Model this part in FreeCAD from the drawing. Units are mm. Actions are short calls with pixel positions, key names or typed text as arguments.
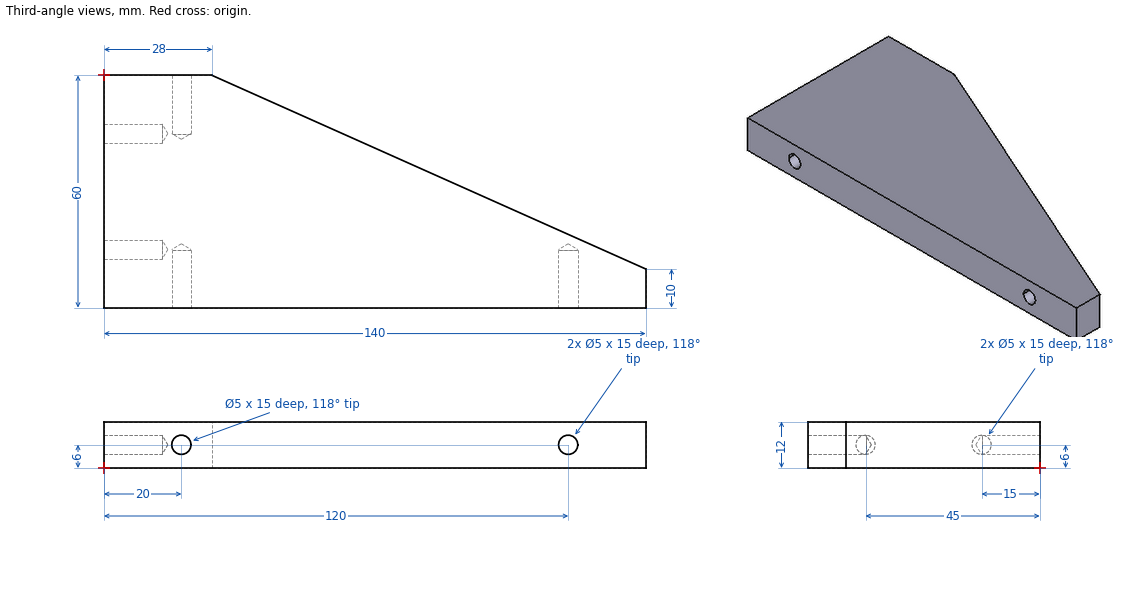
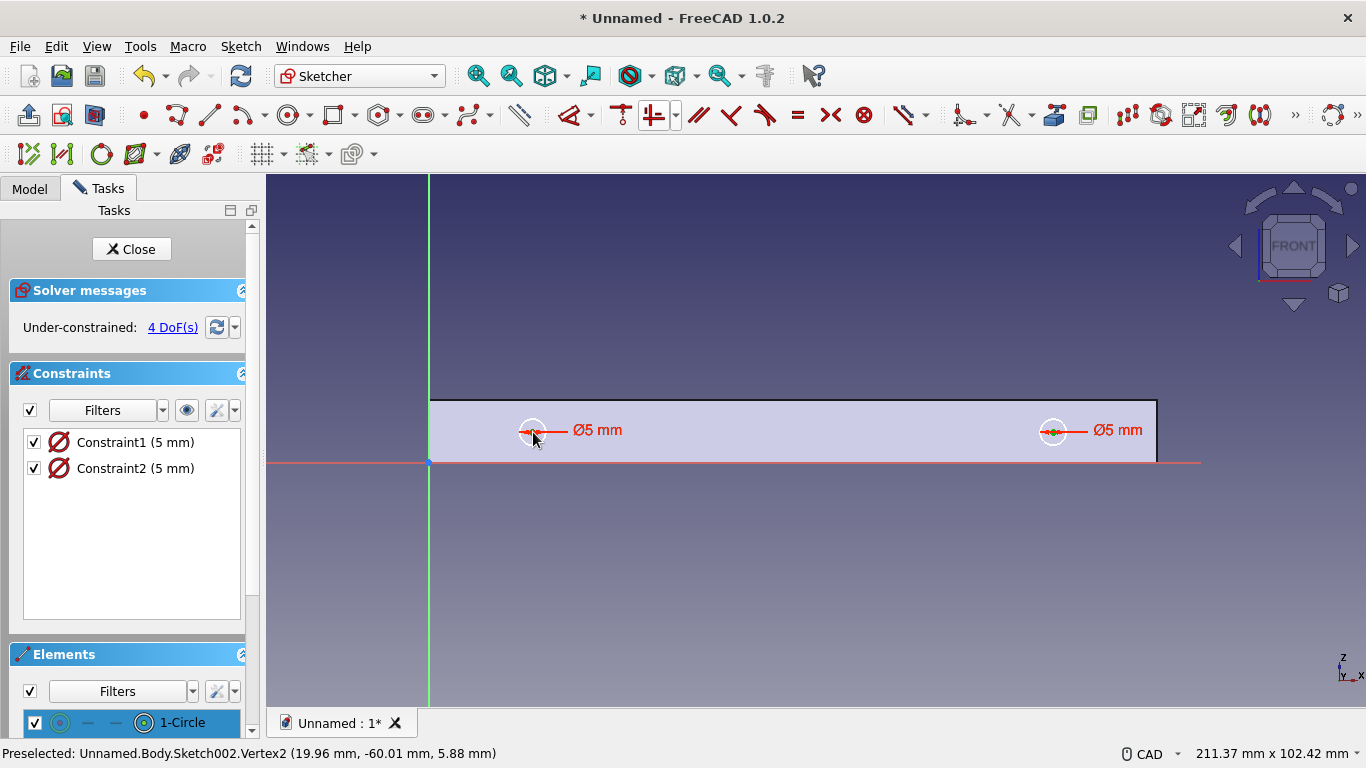
key(h)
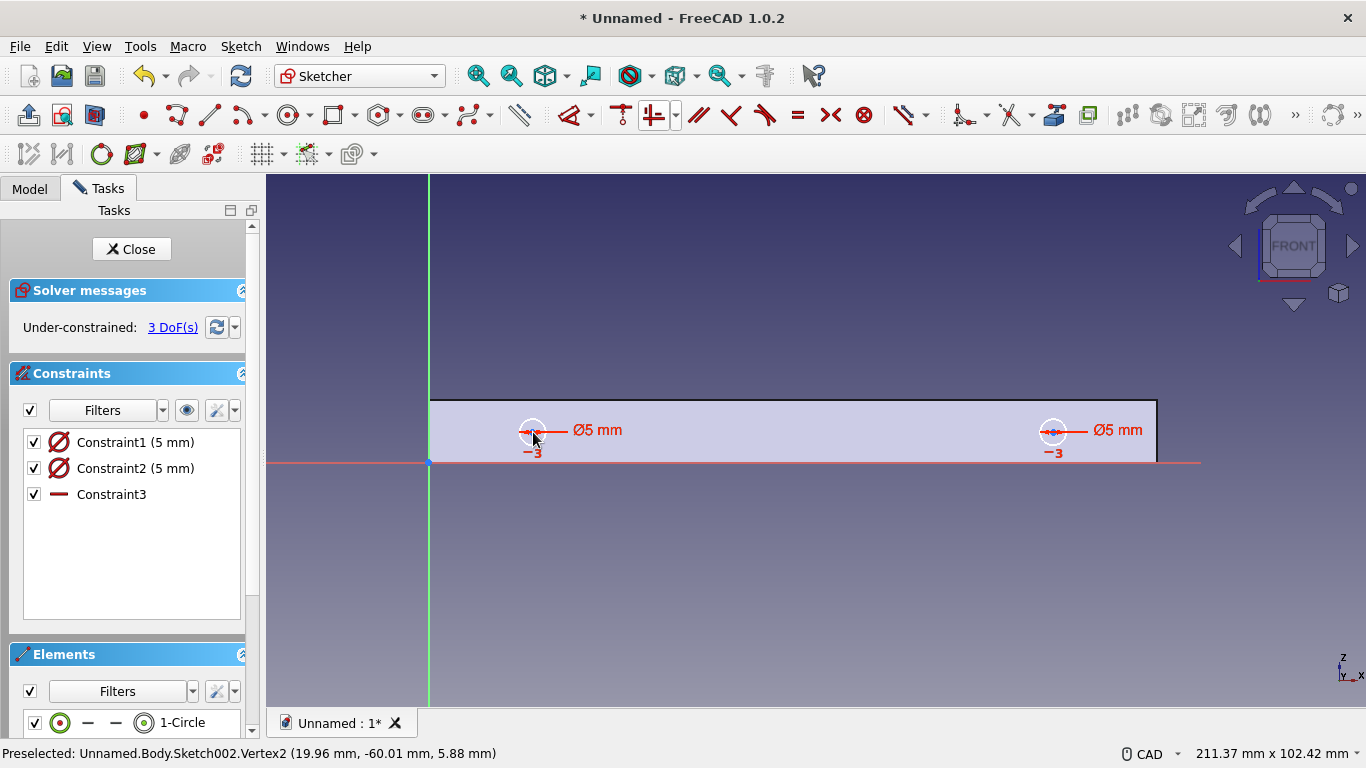
click(568, 116)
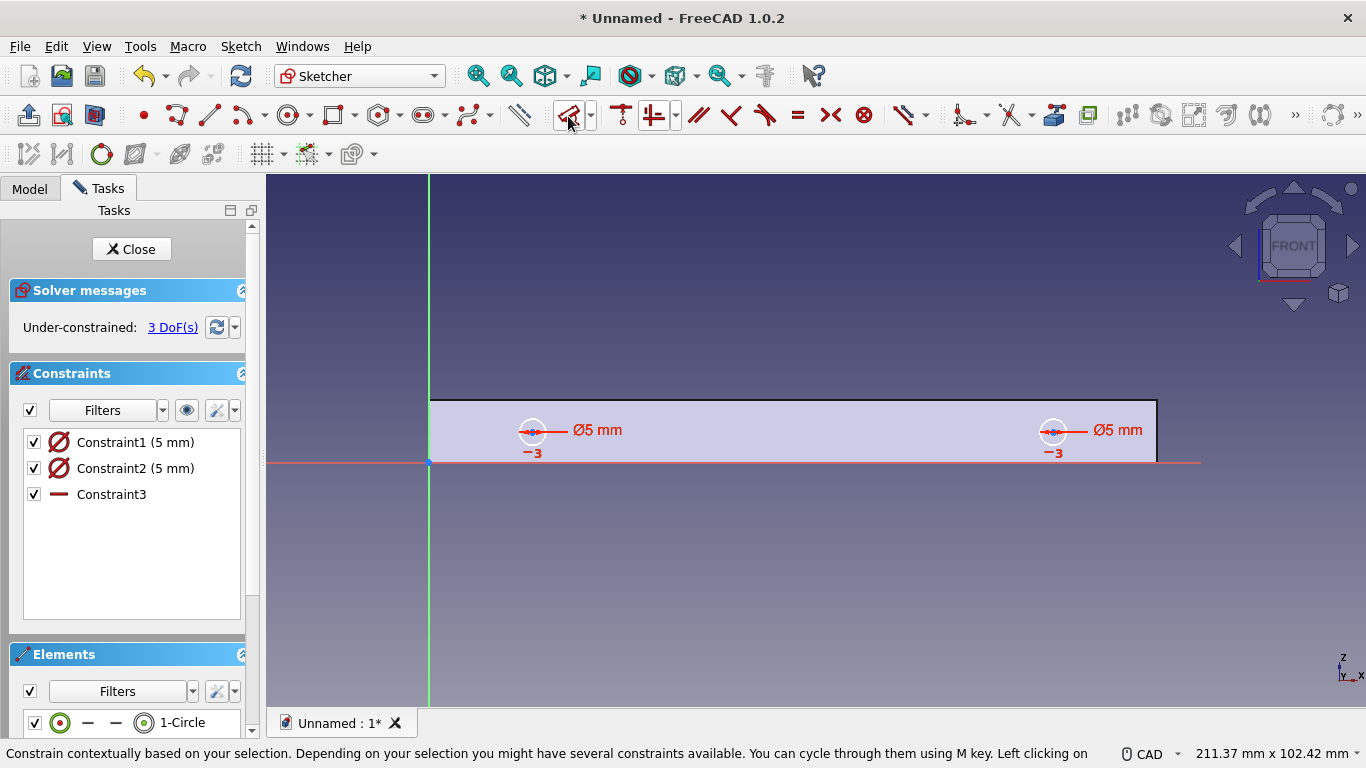
scroll(1053, 432, up, 2)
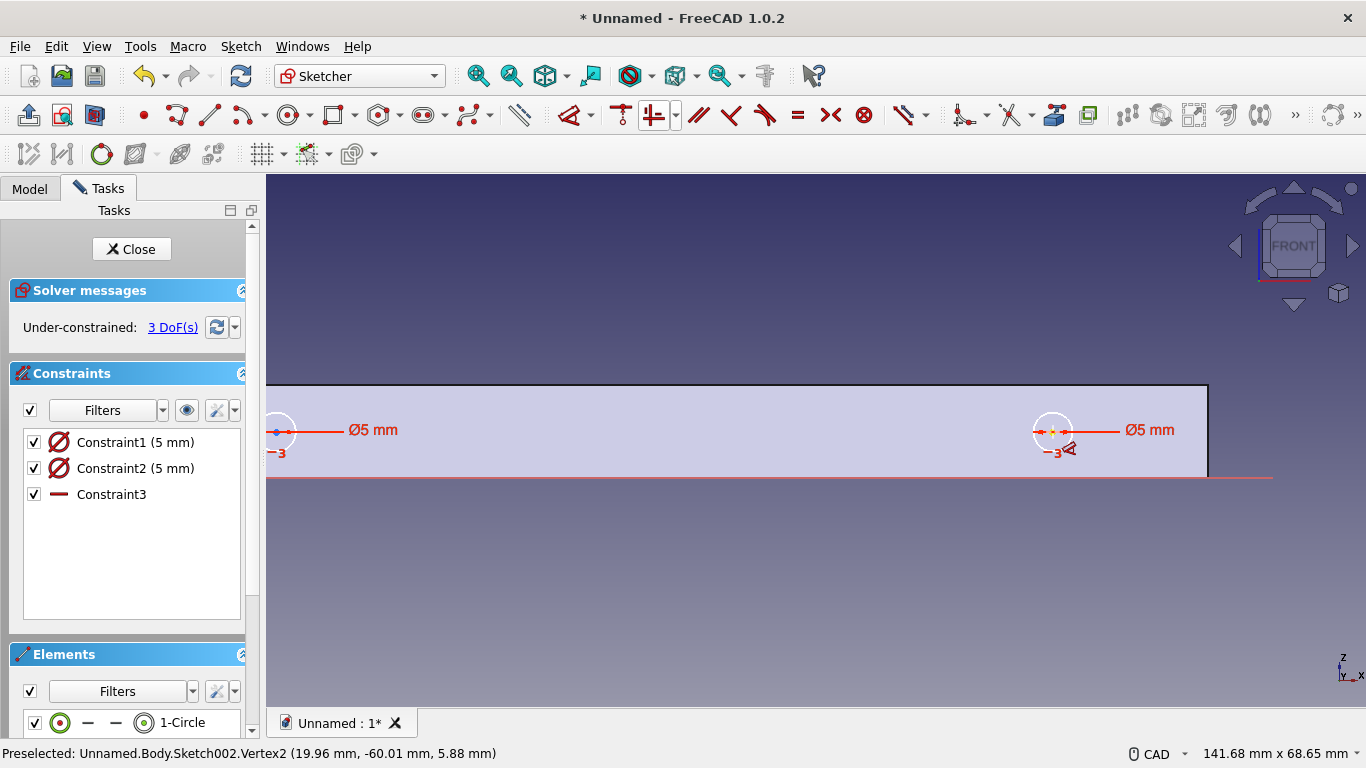
click(1053, 432)
click(1087, 455)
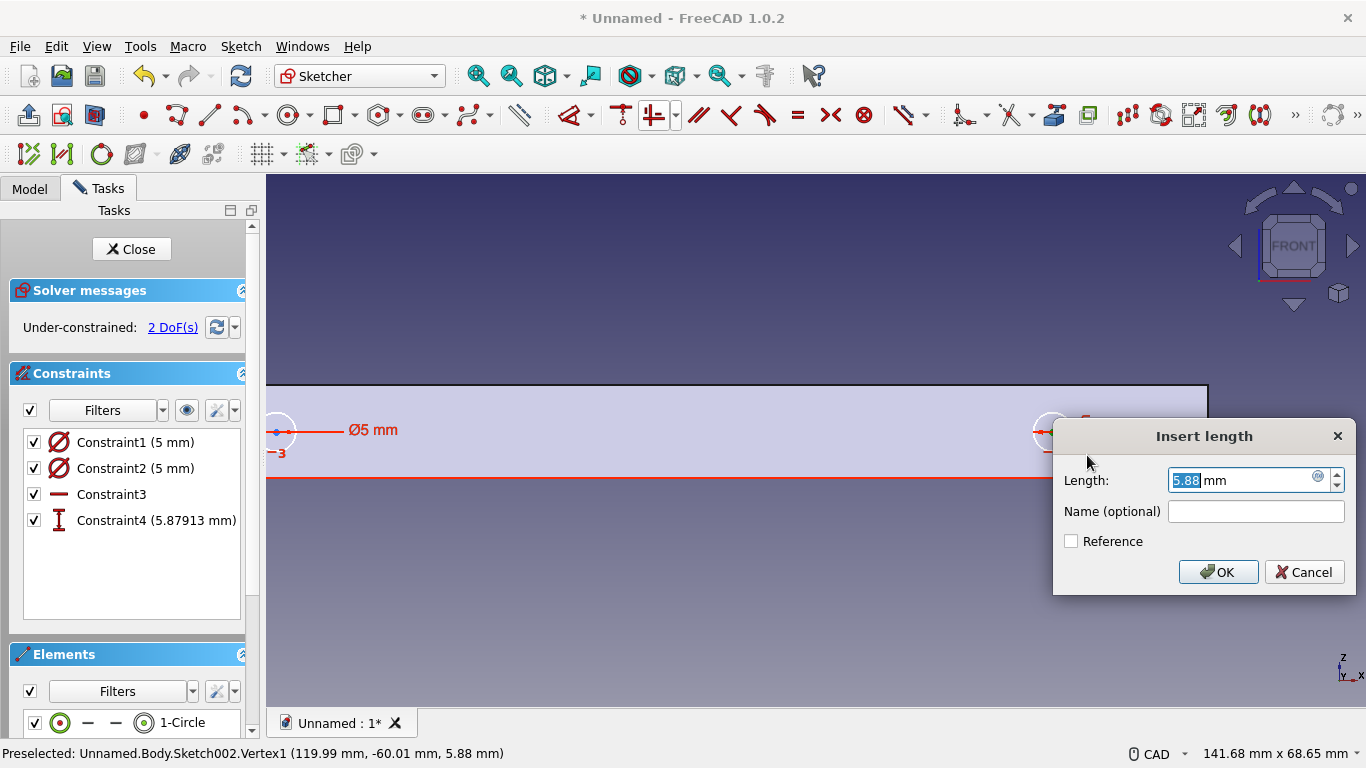
text(6)
key(Return)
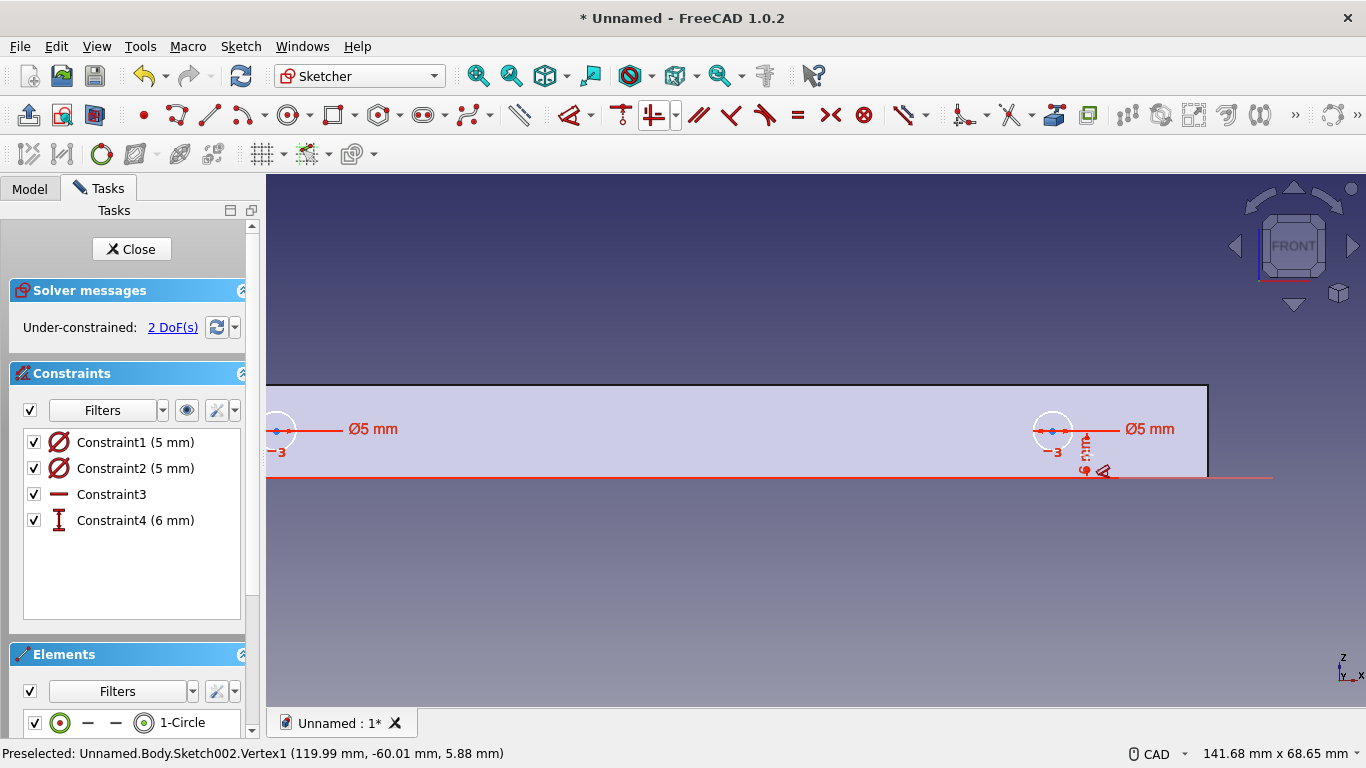
scroll(1054, 432, down, 2)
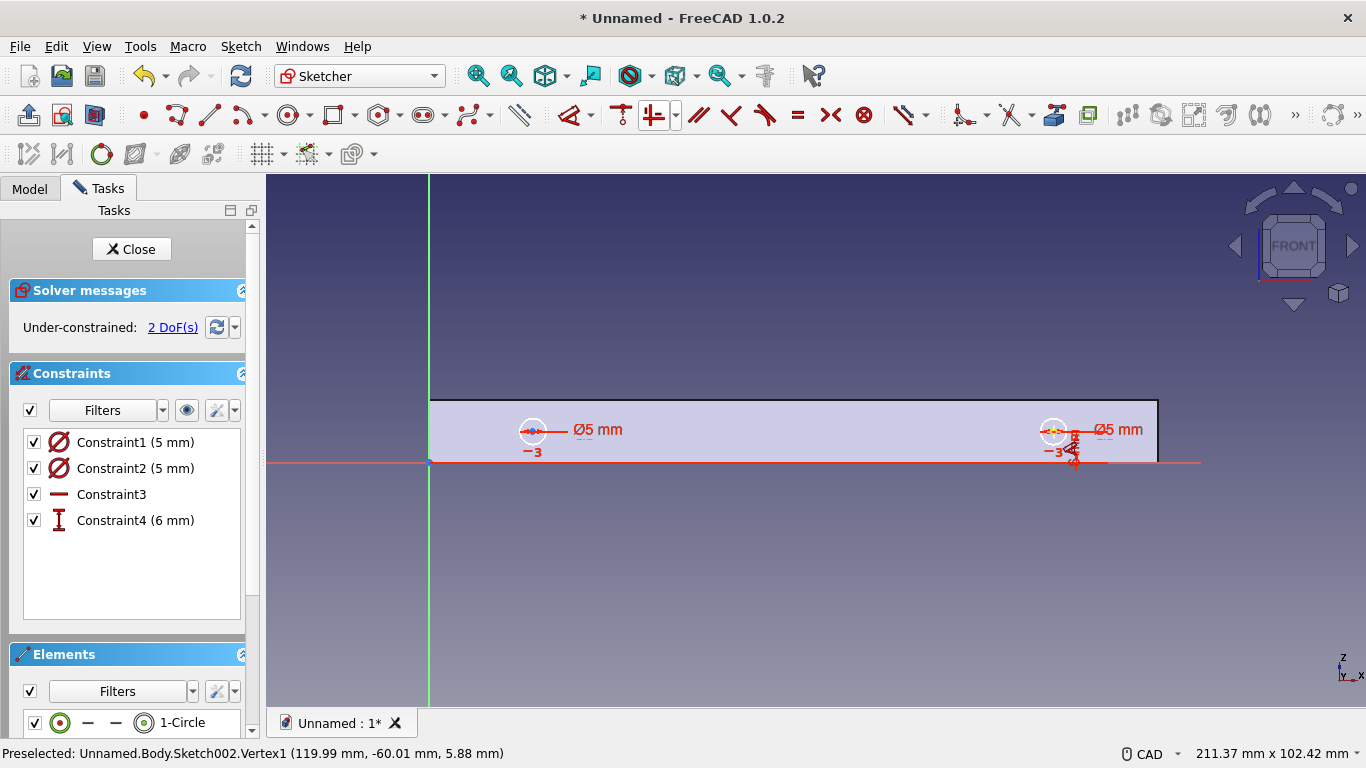
click(533, 432)
click(481, 497)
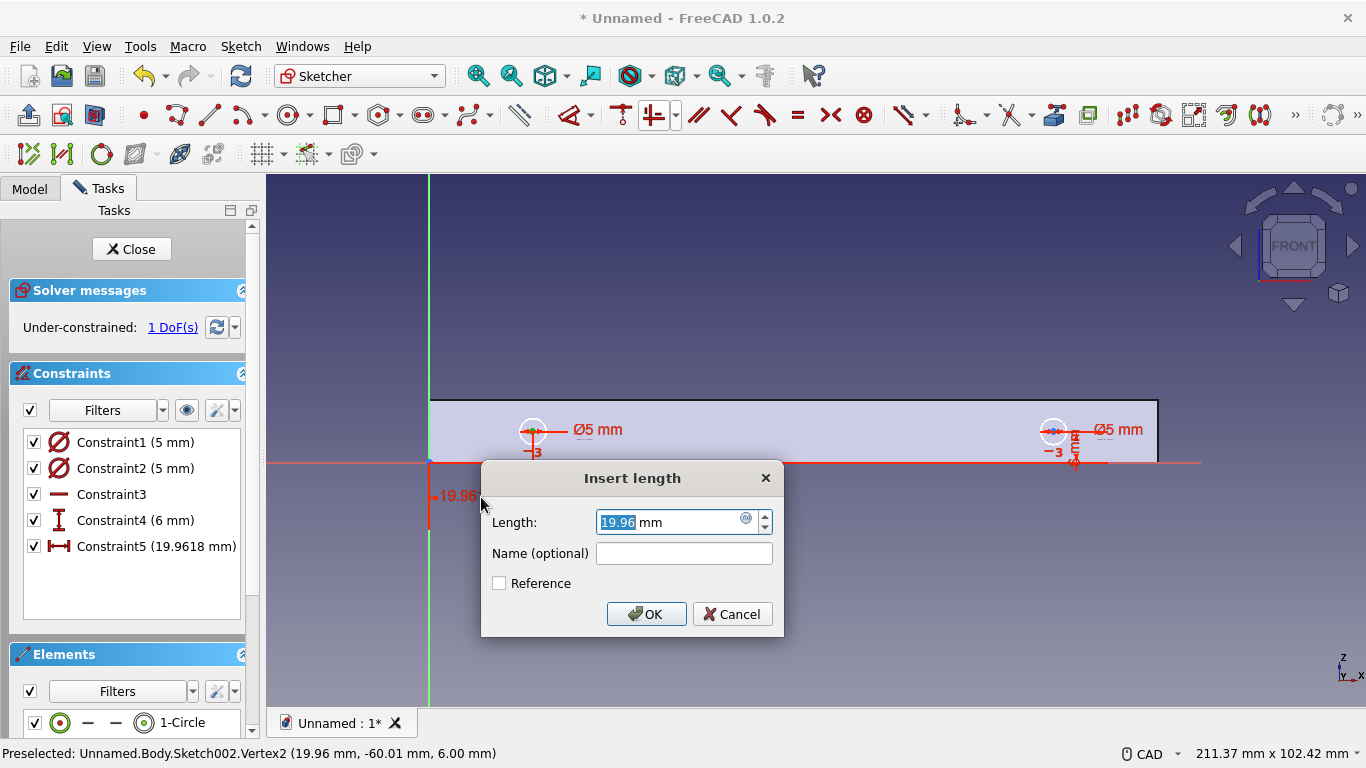
text(20)
key(Return)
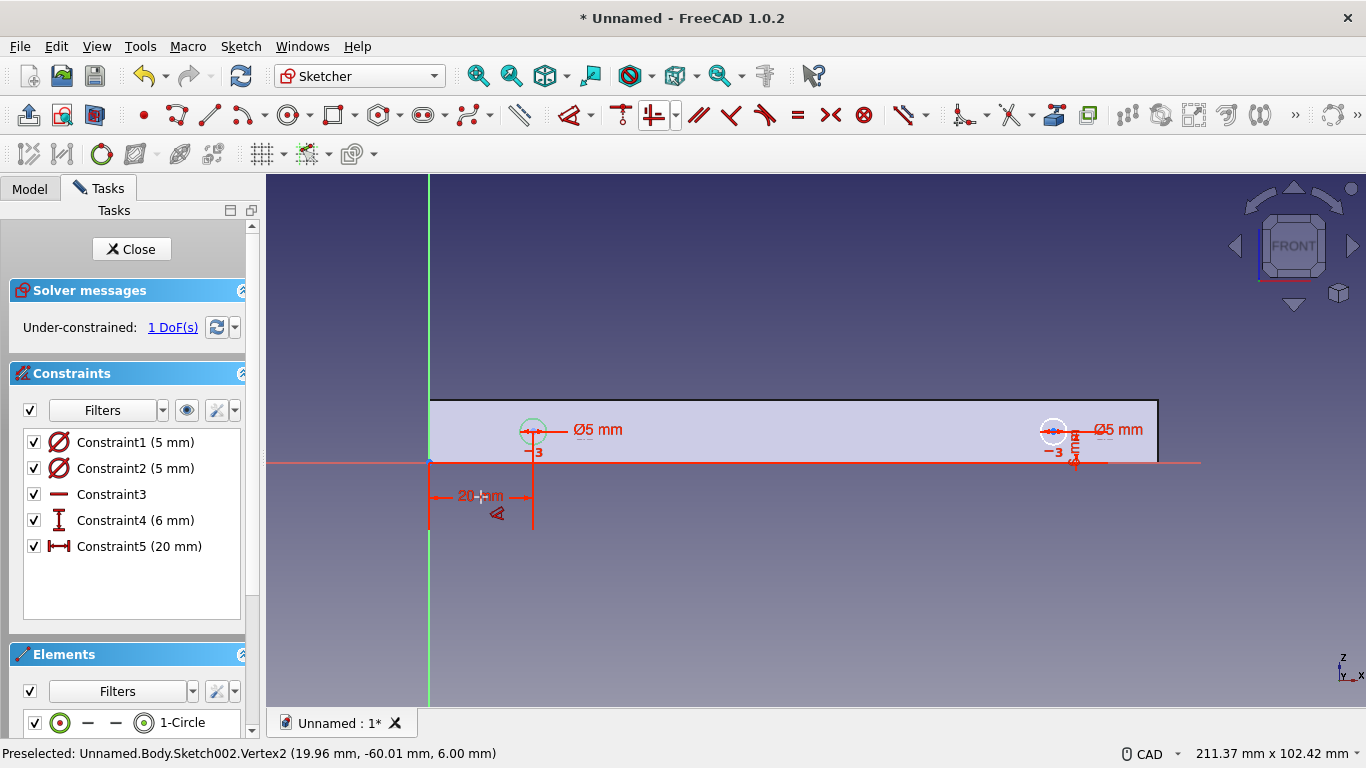
click(1054, 432)
click(741, 497)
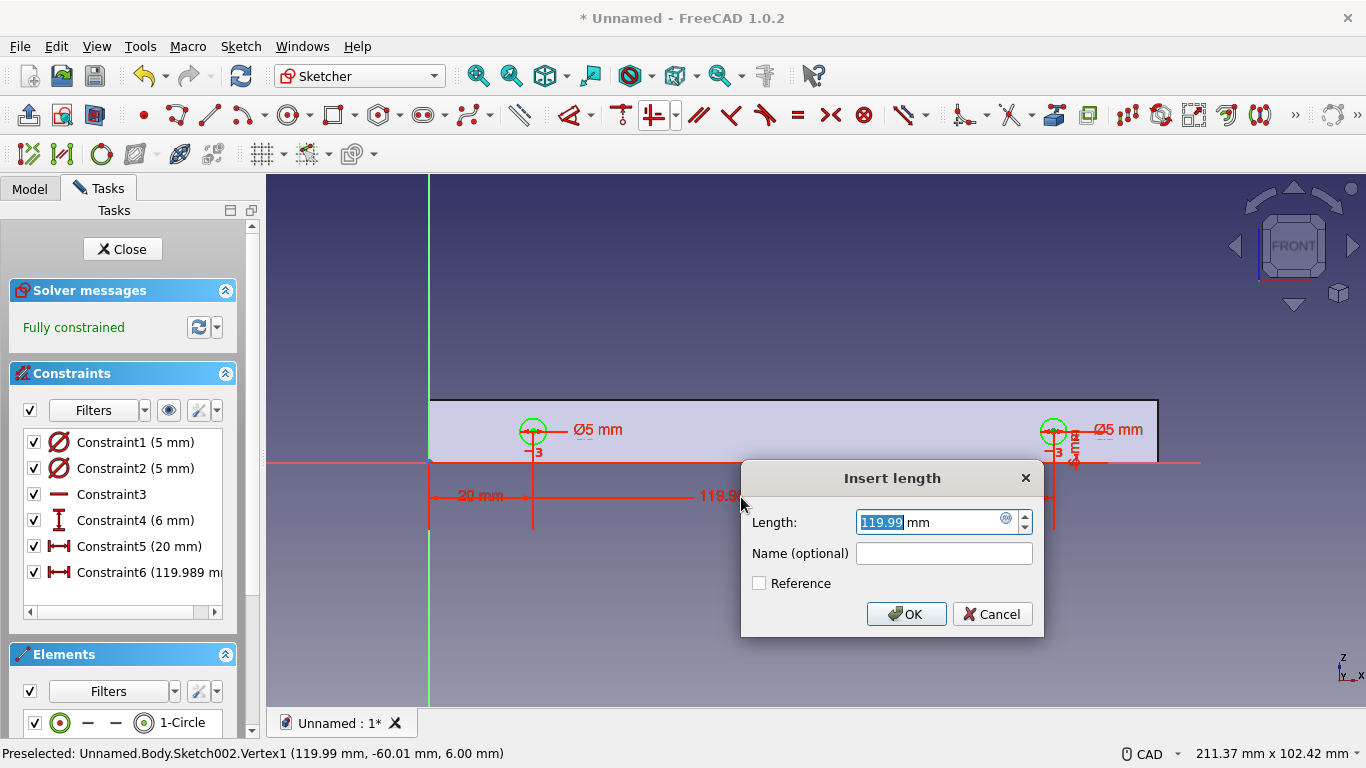
text(120)
key(Return)
key(Escape)